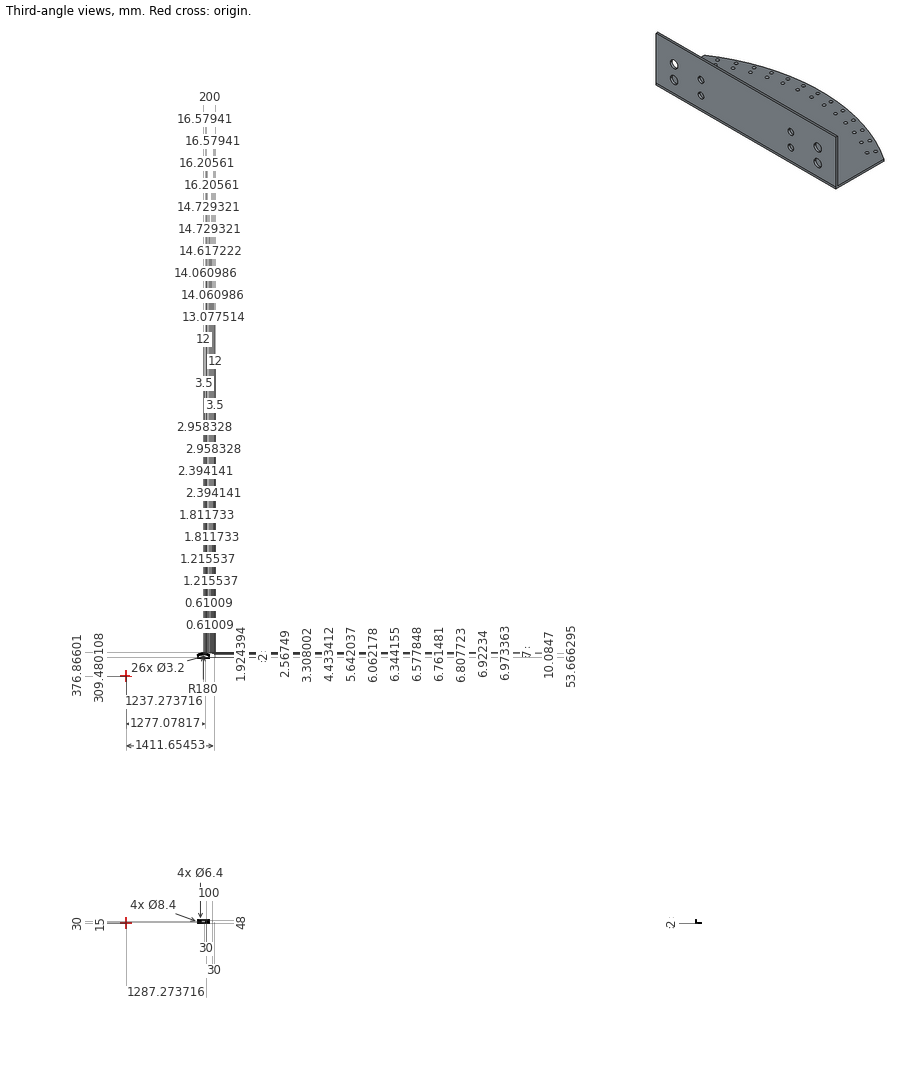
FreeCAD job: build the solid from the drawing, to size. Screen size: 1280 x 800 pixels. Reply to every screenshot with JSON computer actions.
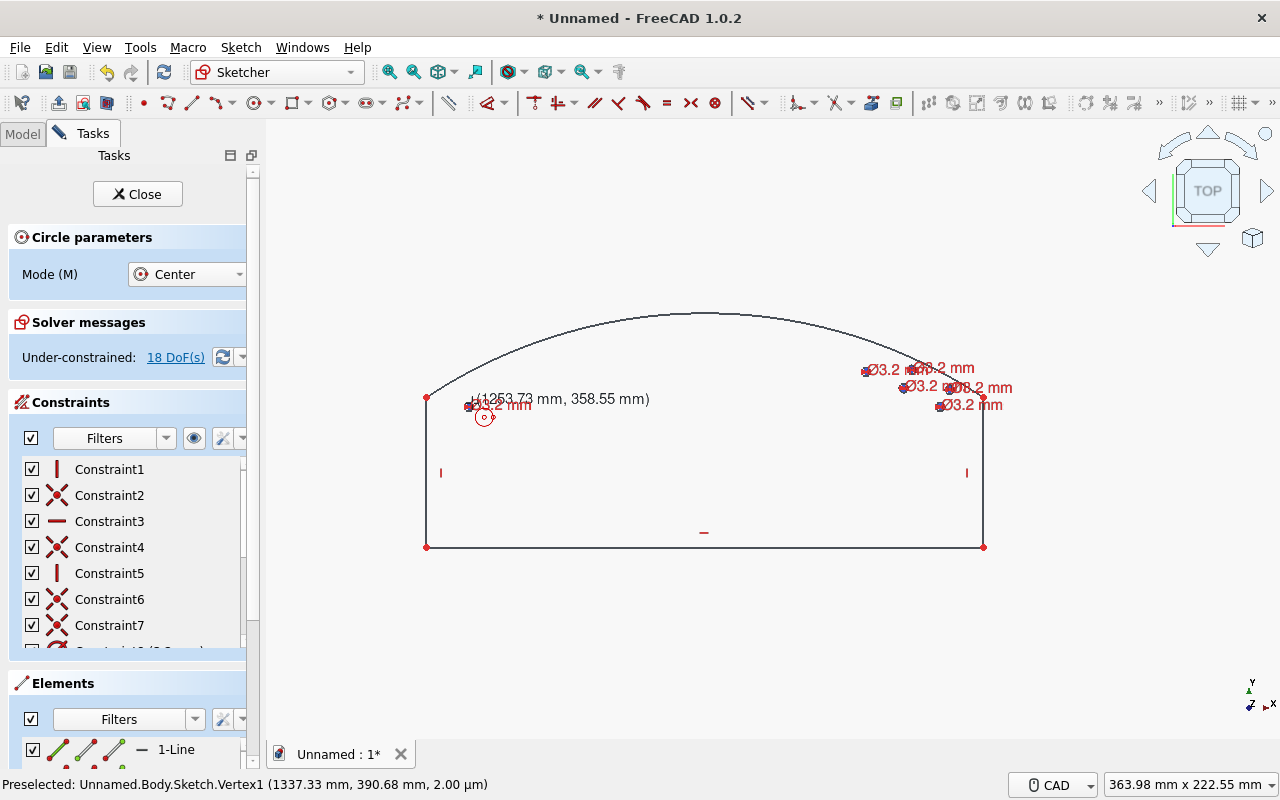
{"action": "scroll", "coordinate": [460, 389], "scroll_direction": "up", "scroll_amount": 9}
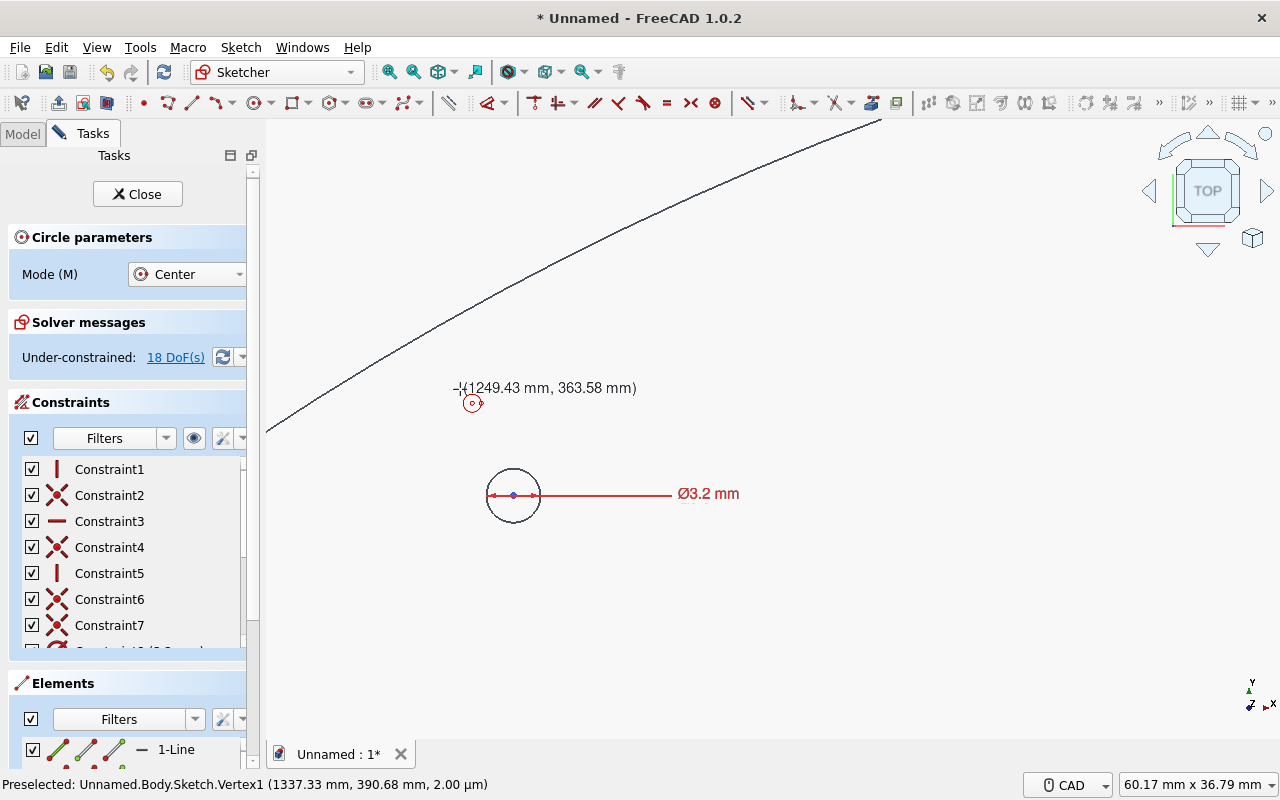
{"action": "scroll", "coordinate": [460, 389], "scroll_direction": "down", "scroll_amount": 9}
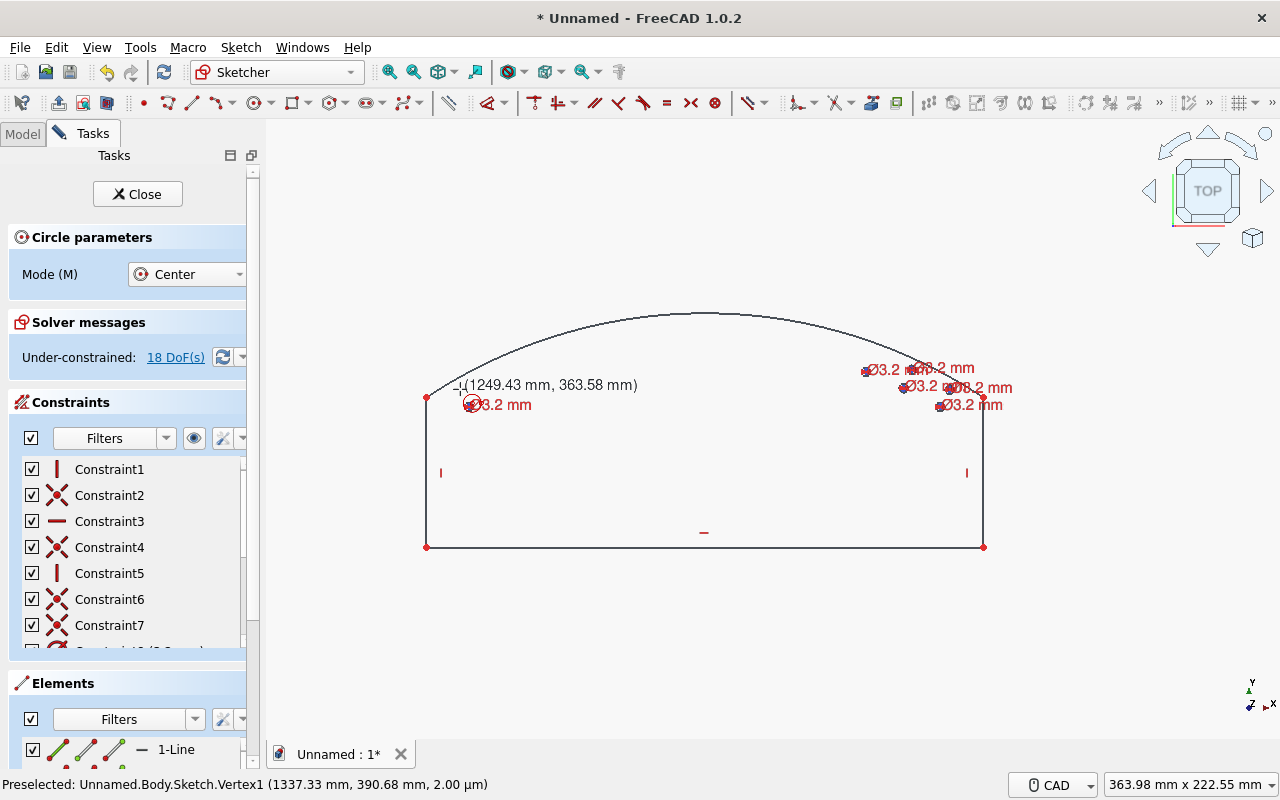
{"action": "scroll", "coordinate": [460, 389], "scroll_direction": "up", "scroll_amount": 2}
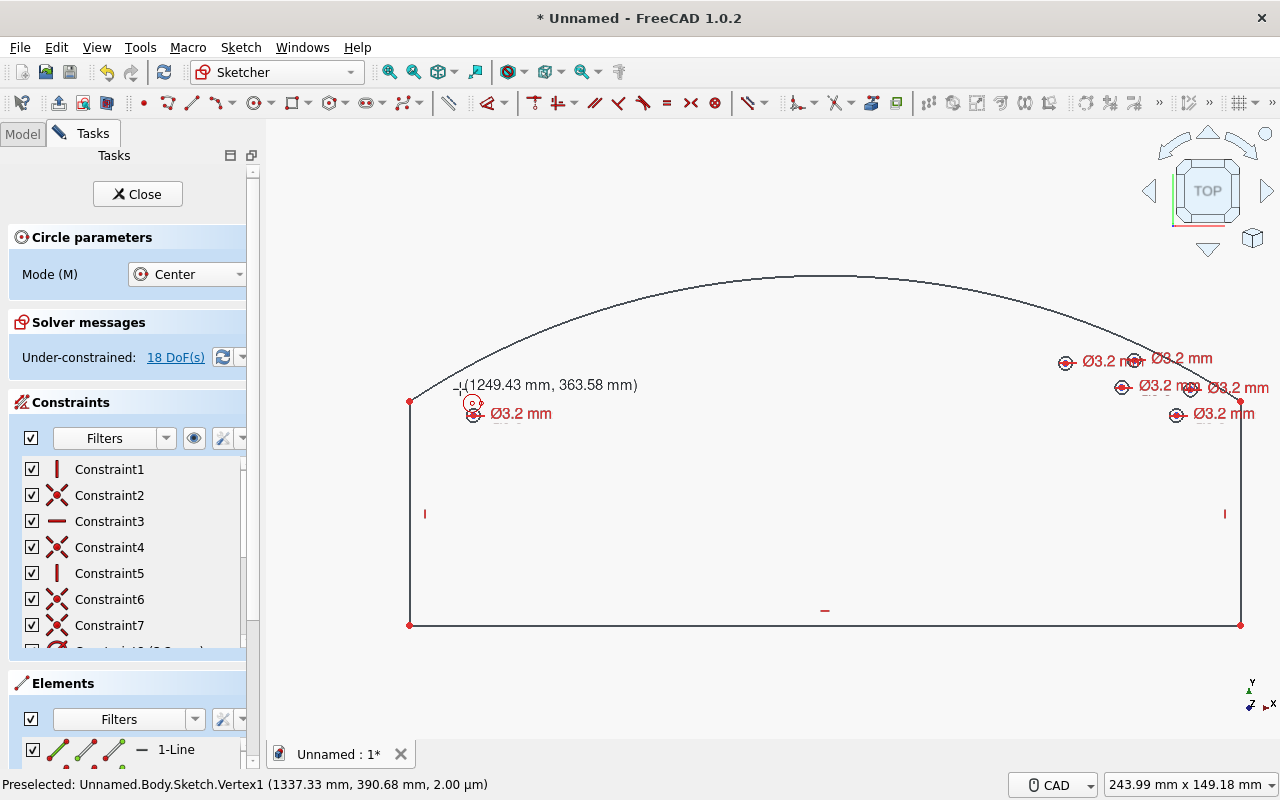
{"action": "left_click", "coordinate": [459, 389]}
{"action": "mouse_move", "coordinate": [464, 384]}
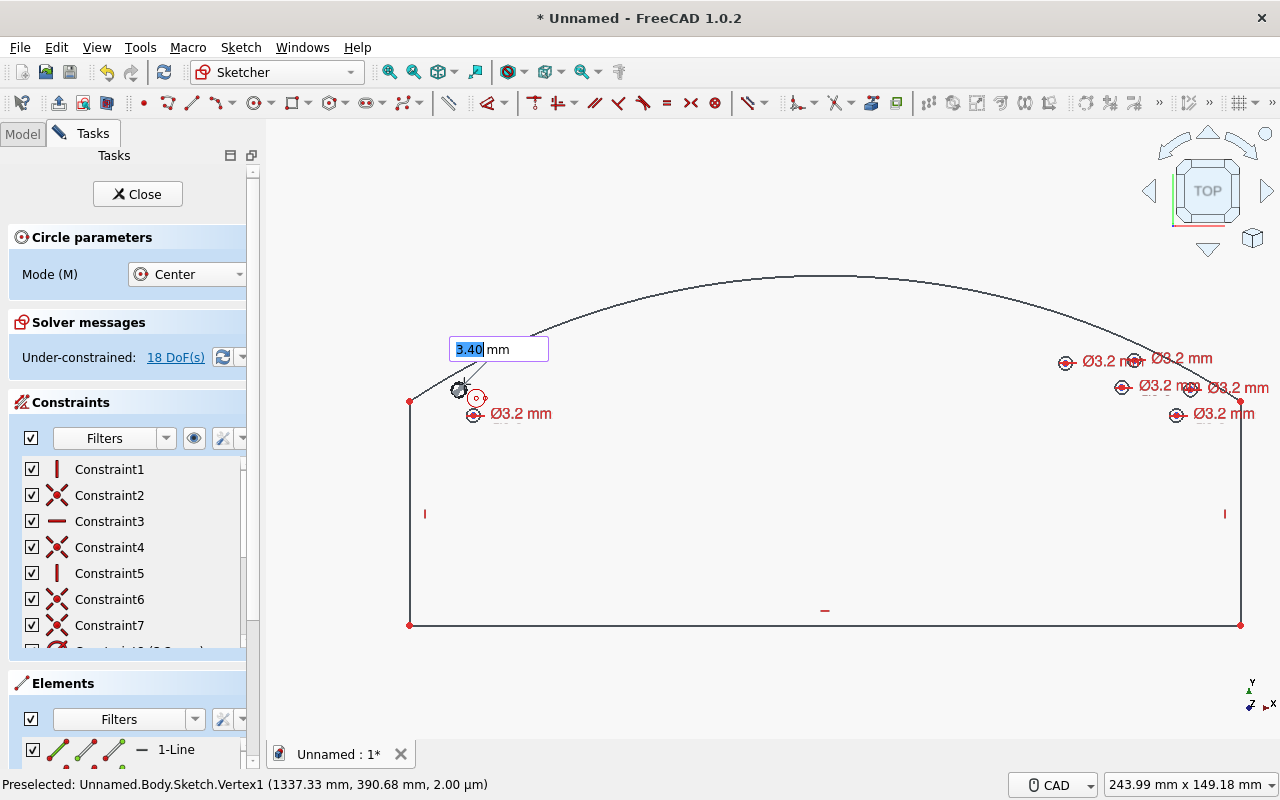
{"action": "type", "text": "3.2"}
{"action": "key", "text": "Return"}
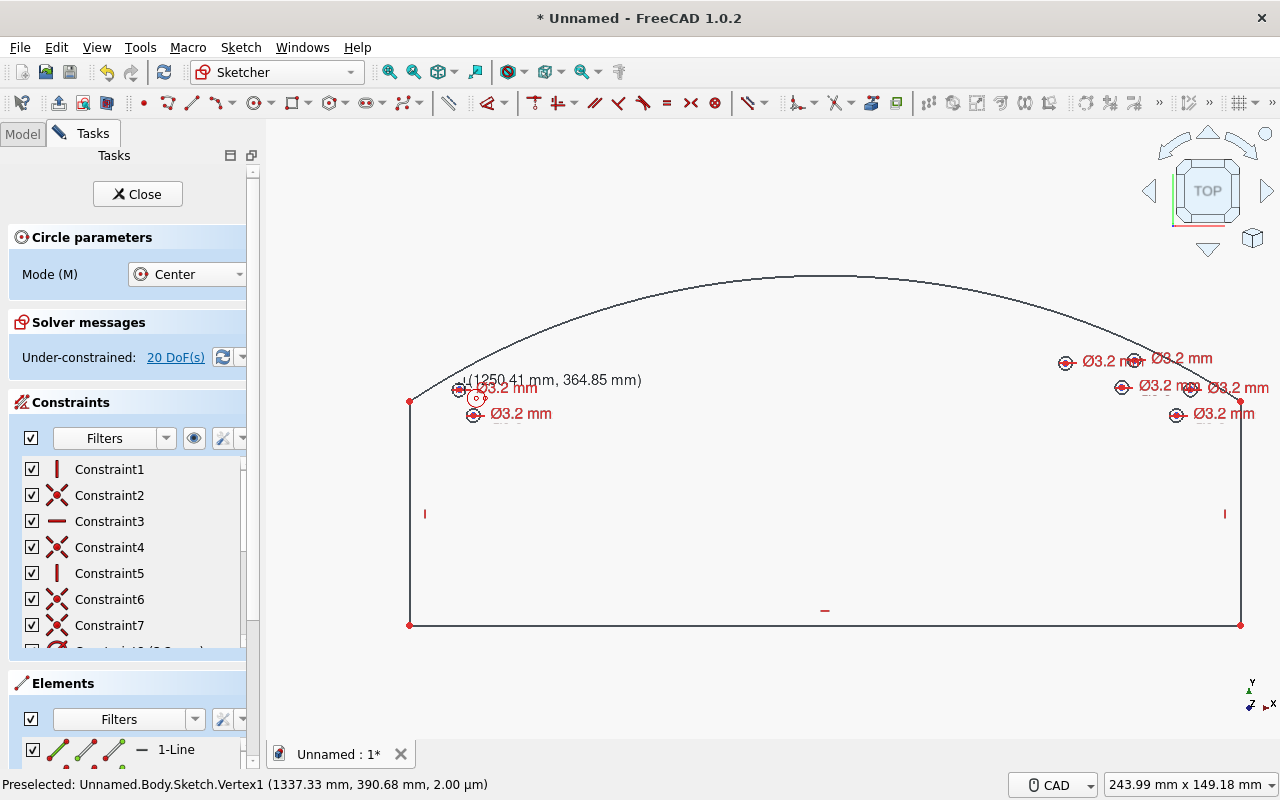
{"action": "scroll", "coordinate": [528, 386], "scroll_direction": "up", "scroll_amount": 7}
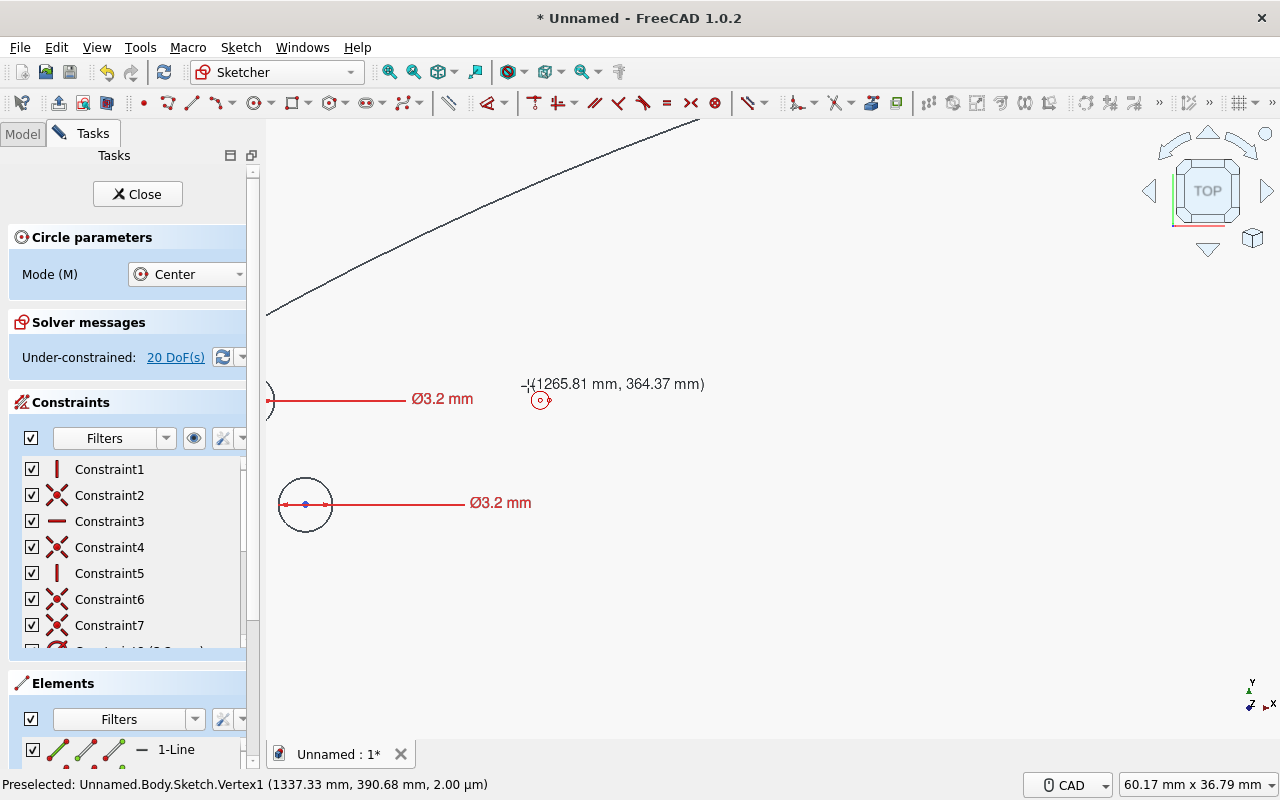
{"action": "scroll", "coordinate": [501, 387], "scroll_direction": "down", "scroll_amount": 9}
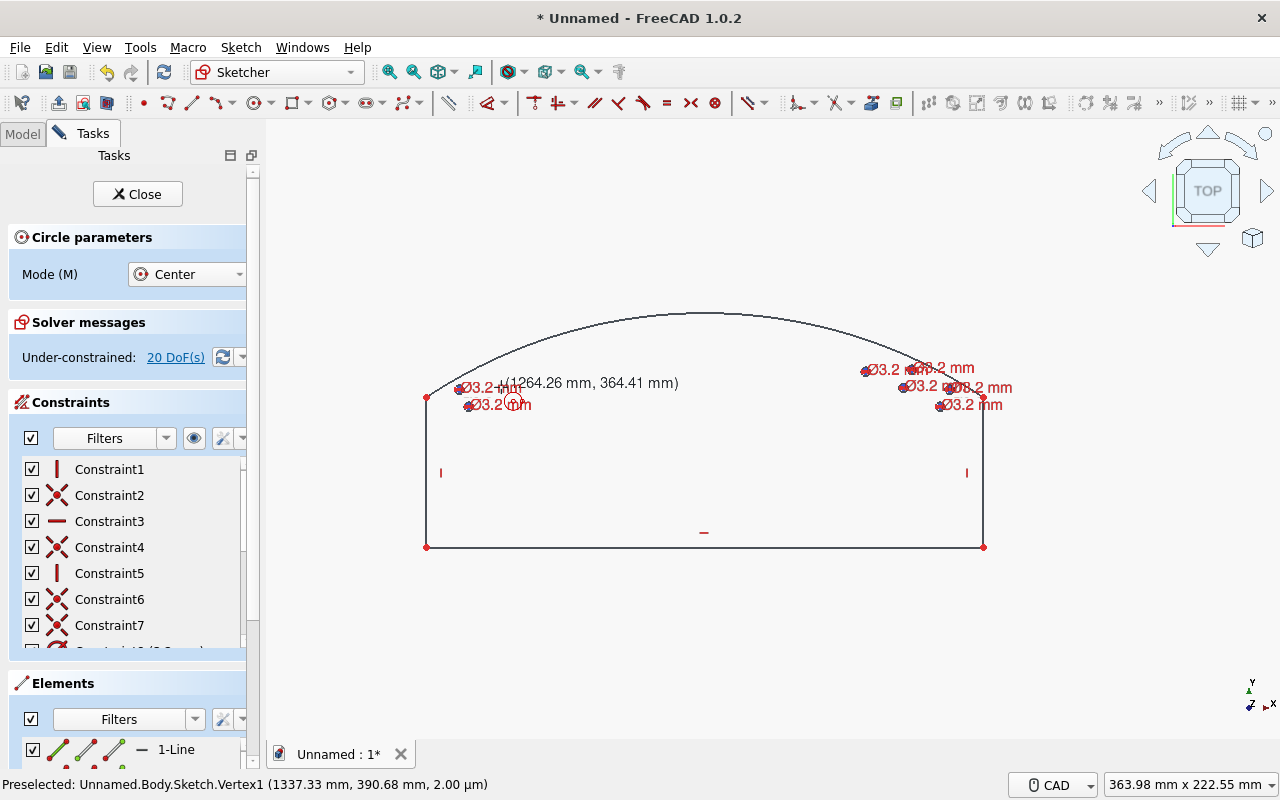
{"action": "left_click", "coordinate": [506, 387]}
{"action": "mouse_move", "coordinate": [509, 384]}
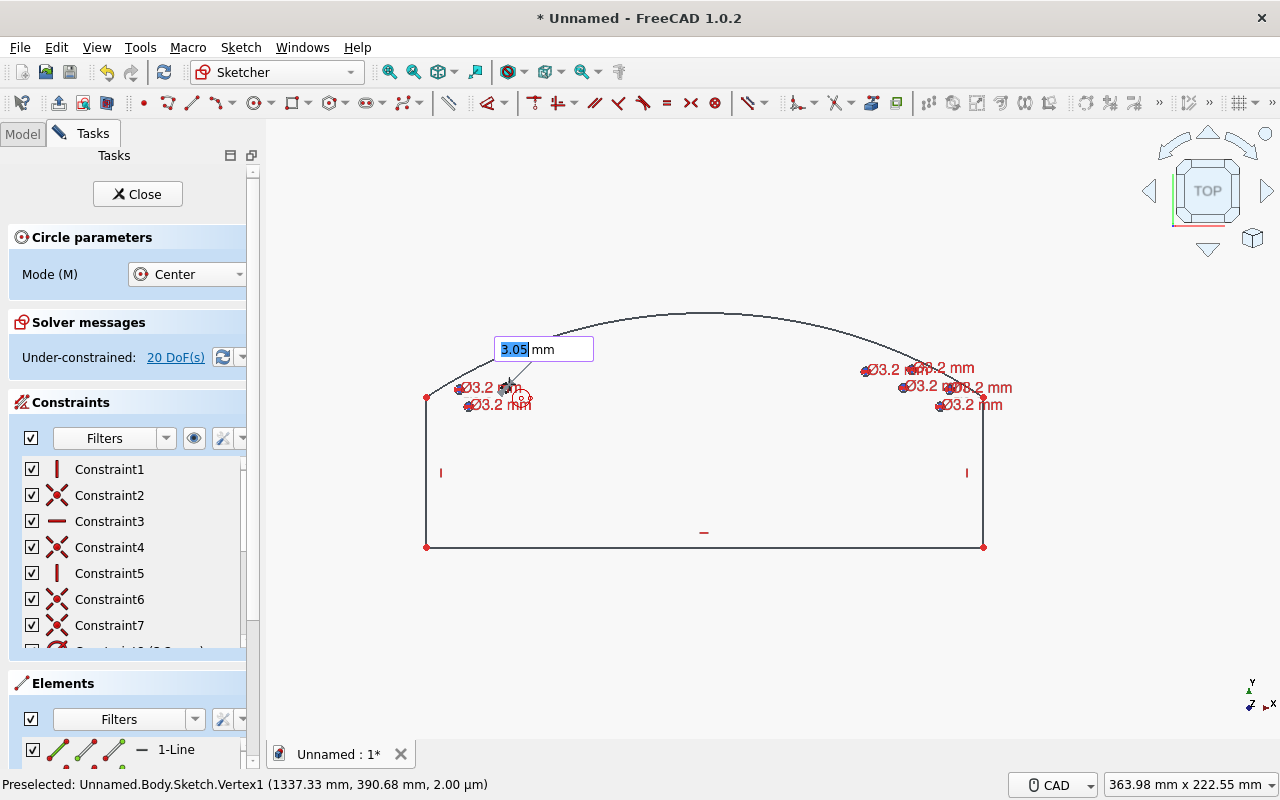
{"action": "type", "text": "3.2"}
{"action": "key", "text": "Return"}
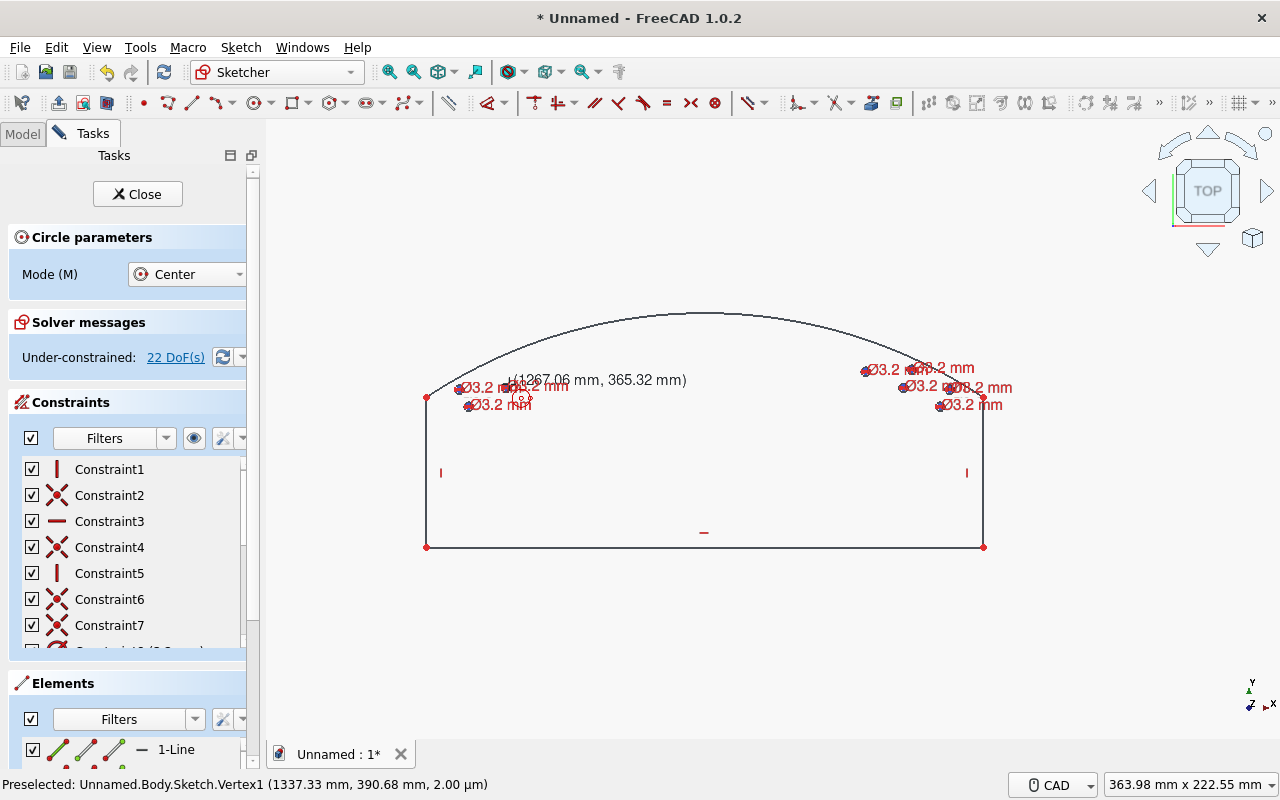
{"action": "scroll", "coordinate": [544, 371], "scroll_direction": "up", "scroll_amount": 9}